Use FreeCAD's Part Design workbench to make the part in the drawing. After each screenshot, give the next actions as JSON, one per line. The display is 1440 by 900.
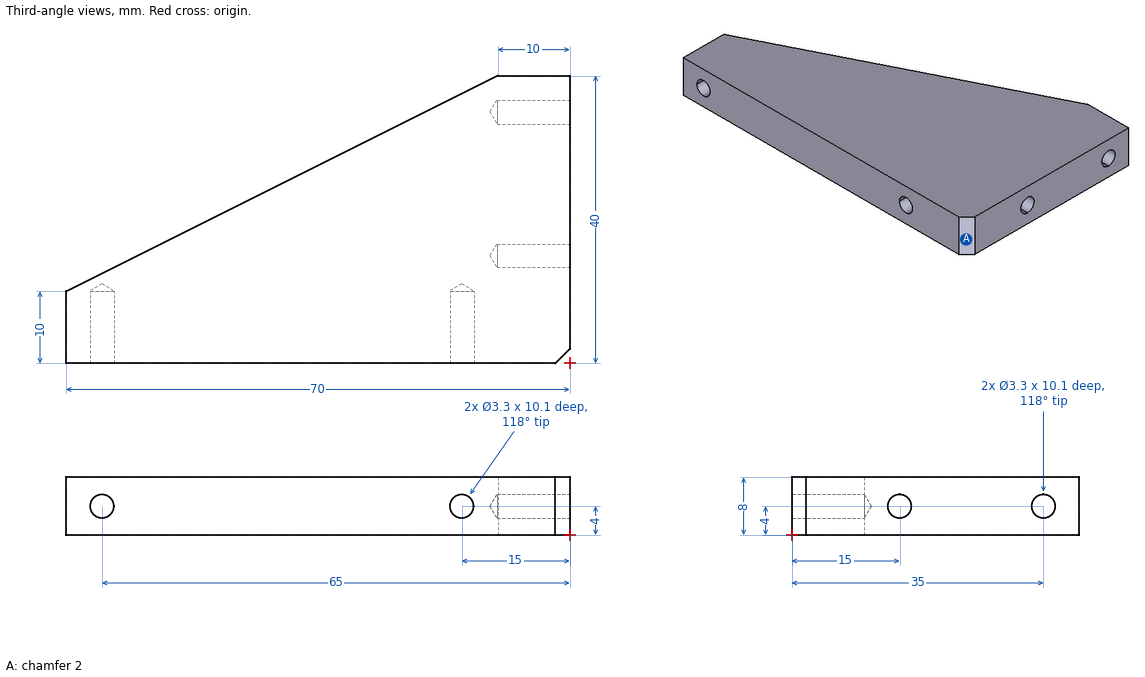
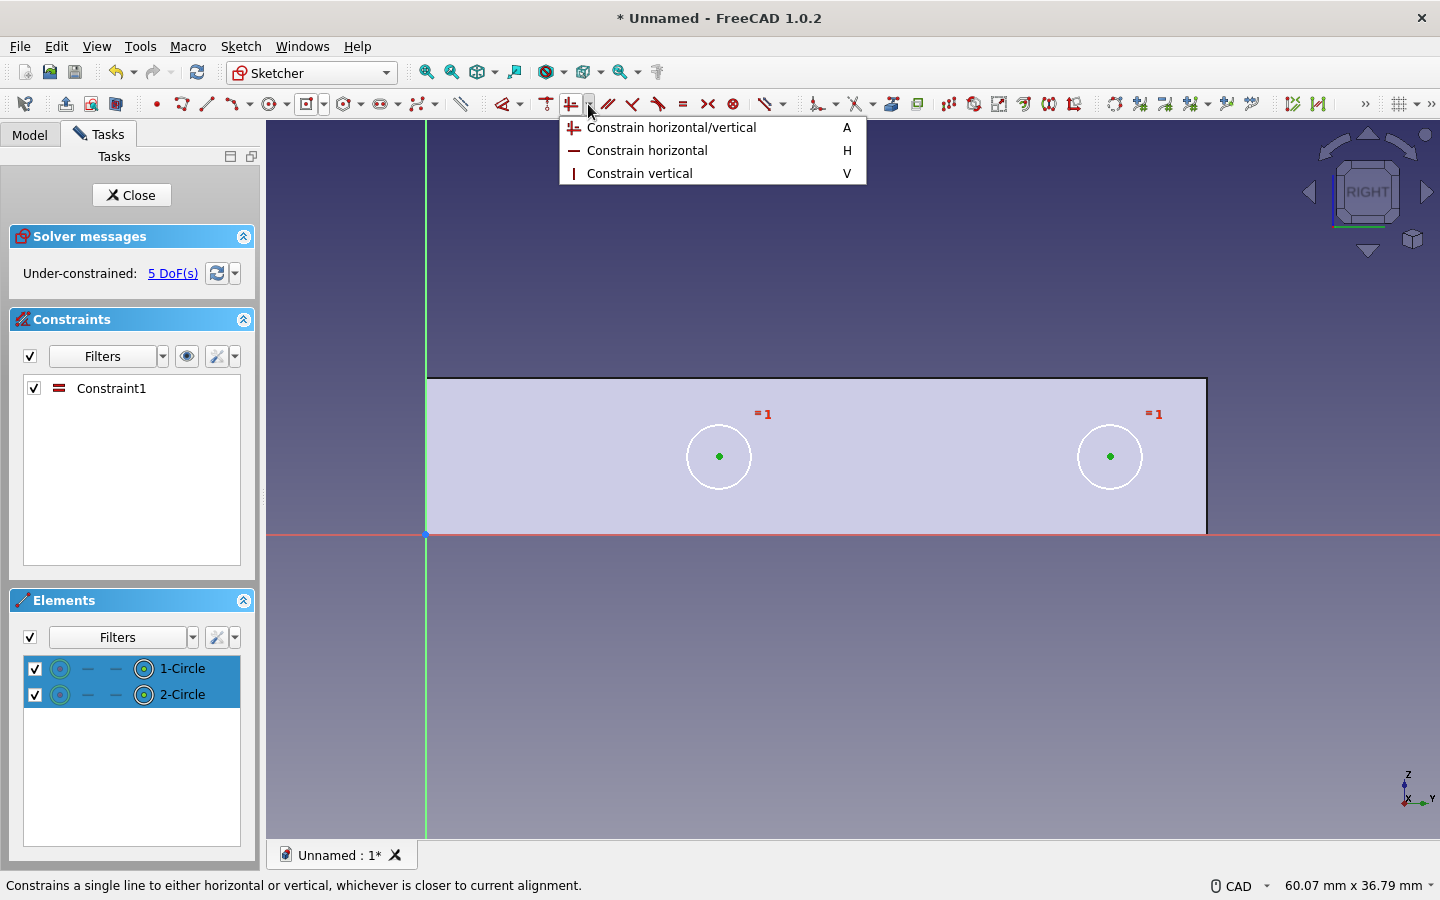
{"action": "left_click", "coordinate": [713, 150]}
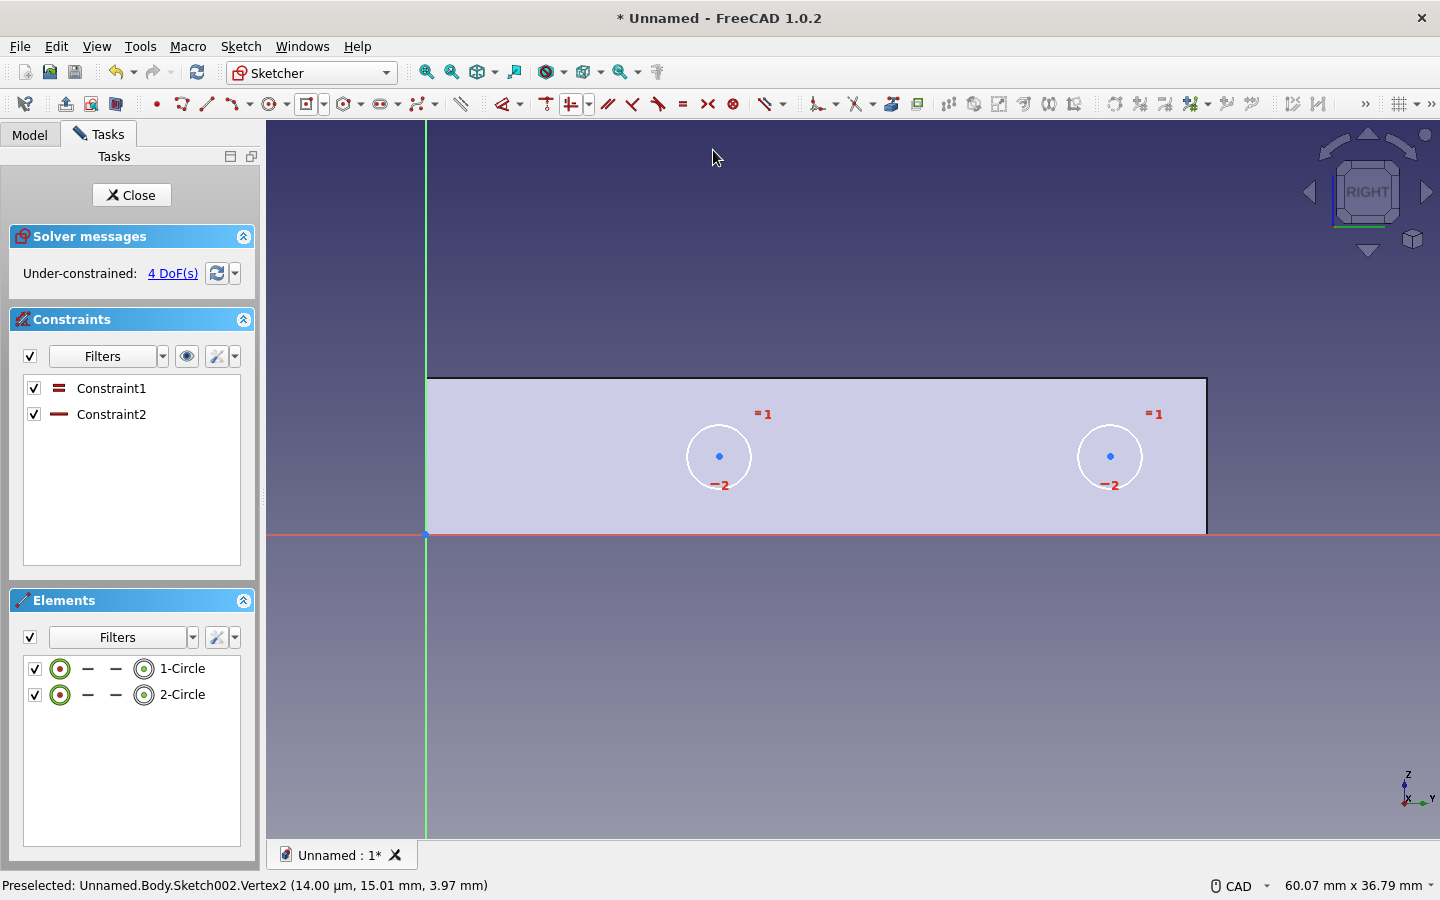
{"action": "left_click", "coordinate": [502, 104]}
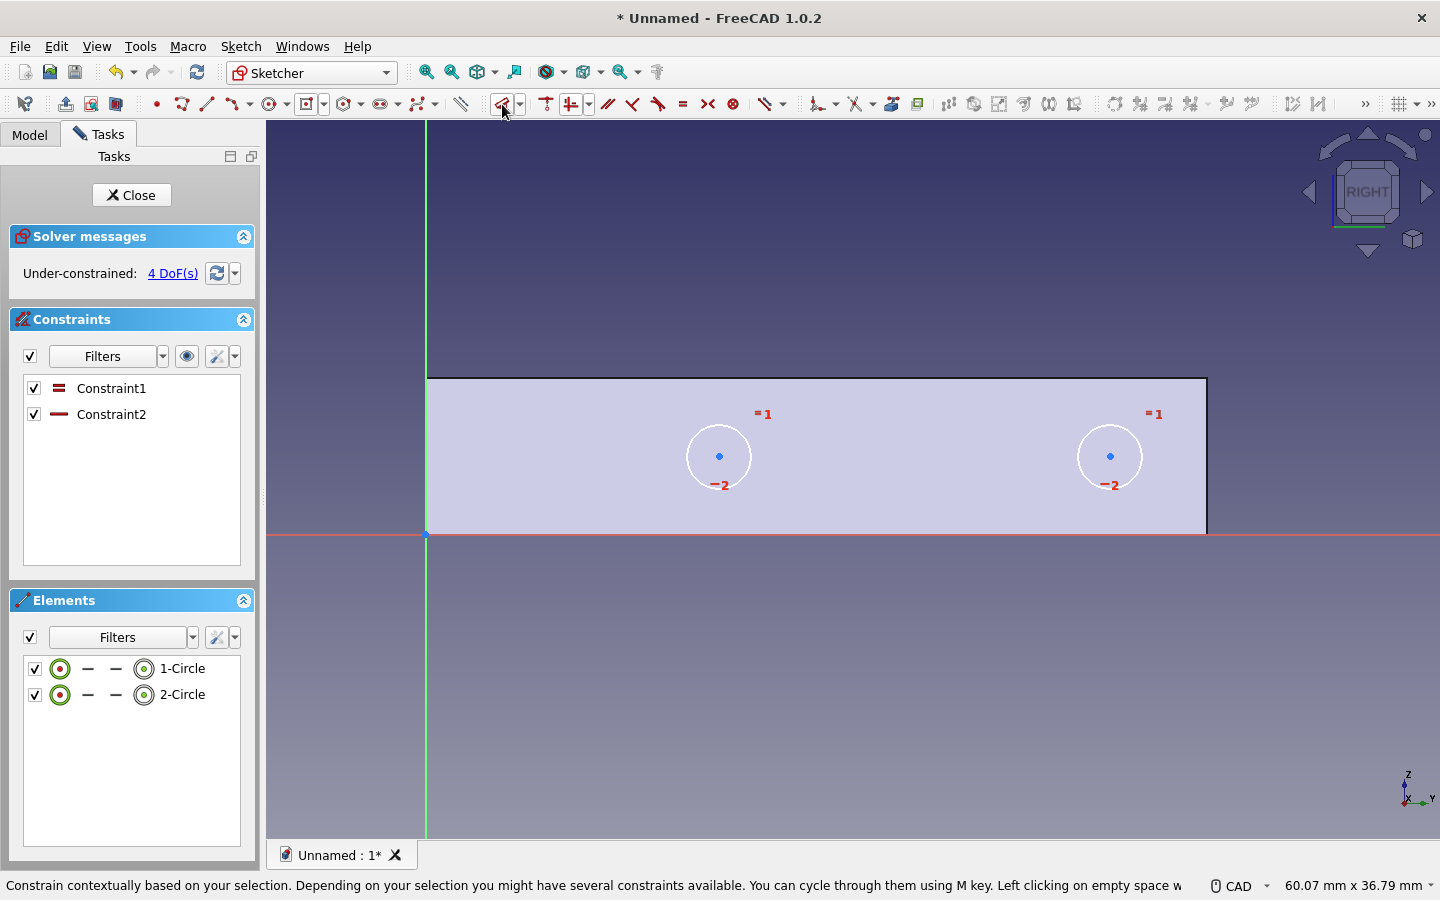
{"action": "left_click", "coordinate": [1132, 434]}
{"action": "left_click", "coordinate": [1154, 411]}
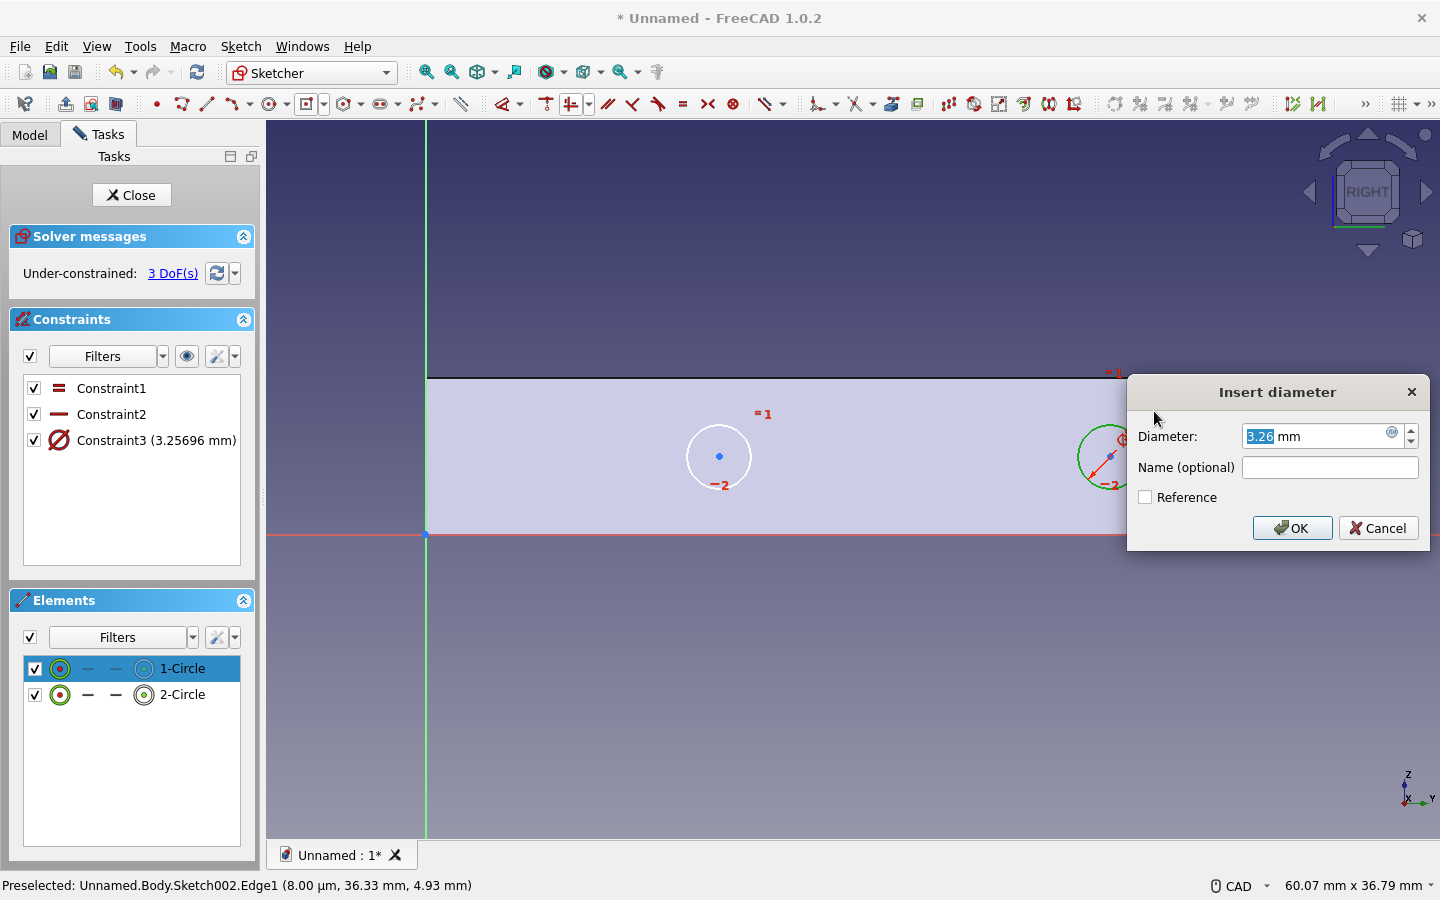
{"action": "type", "text": "3.3"}
{"action": "key", "text": "Return"}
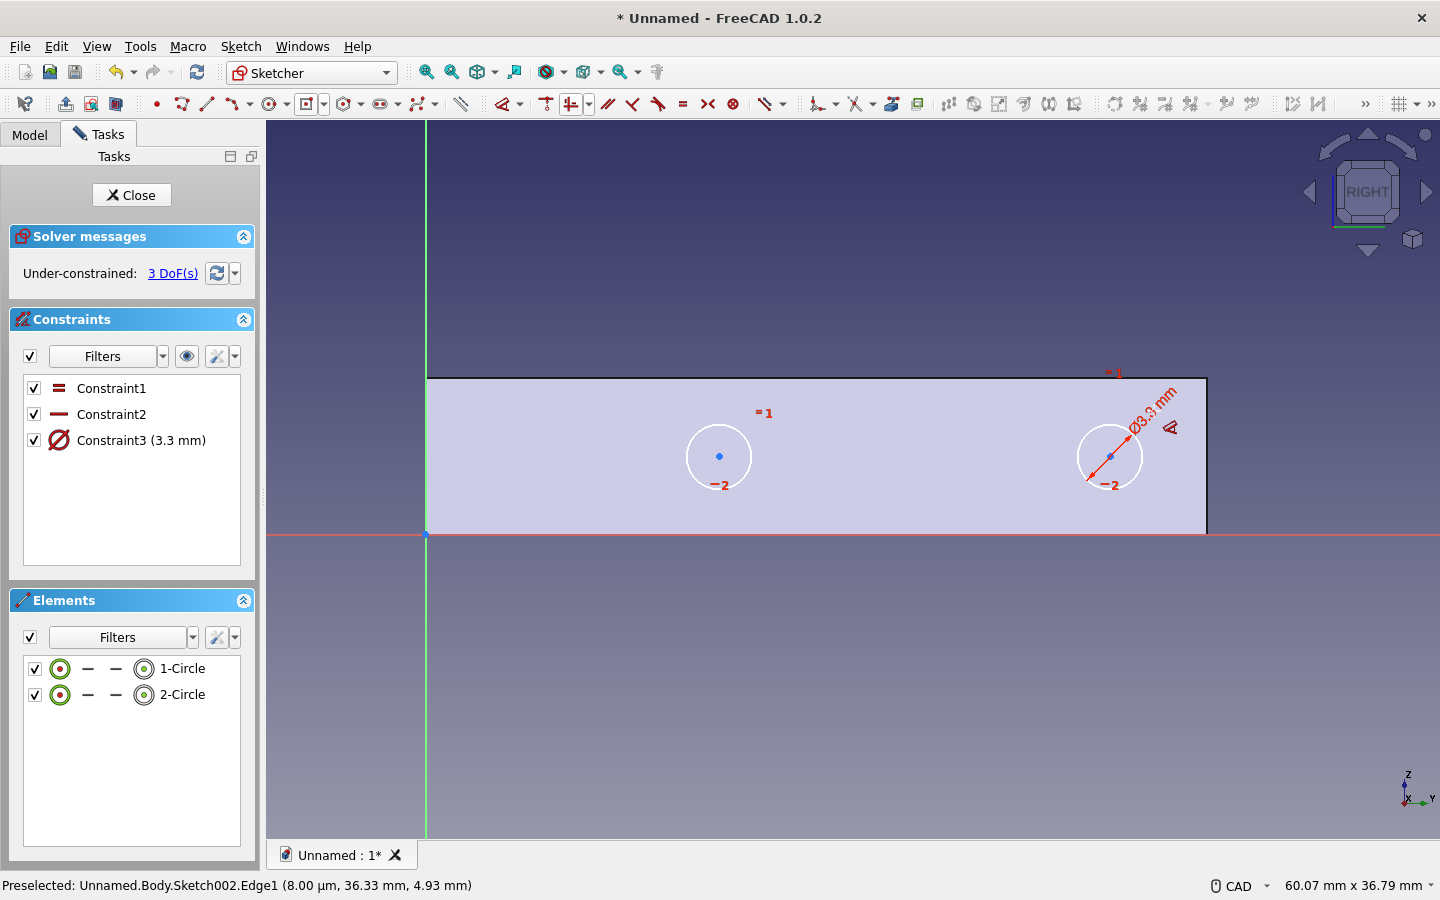
{"action": "left_click", "coordinate": [1110, 457]}
{"action": "left_click", "coordinate": [392, 496]}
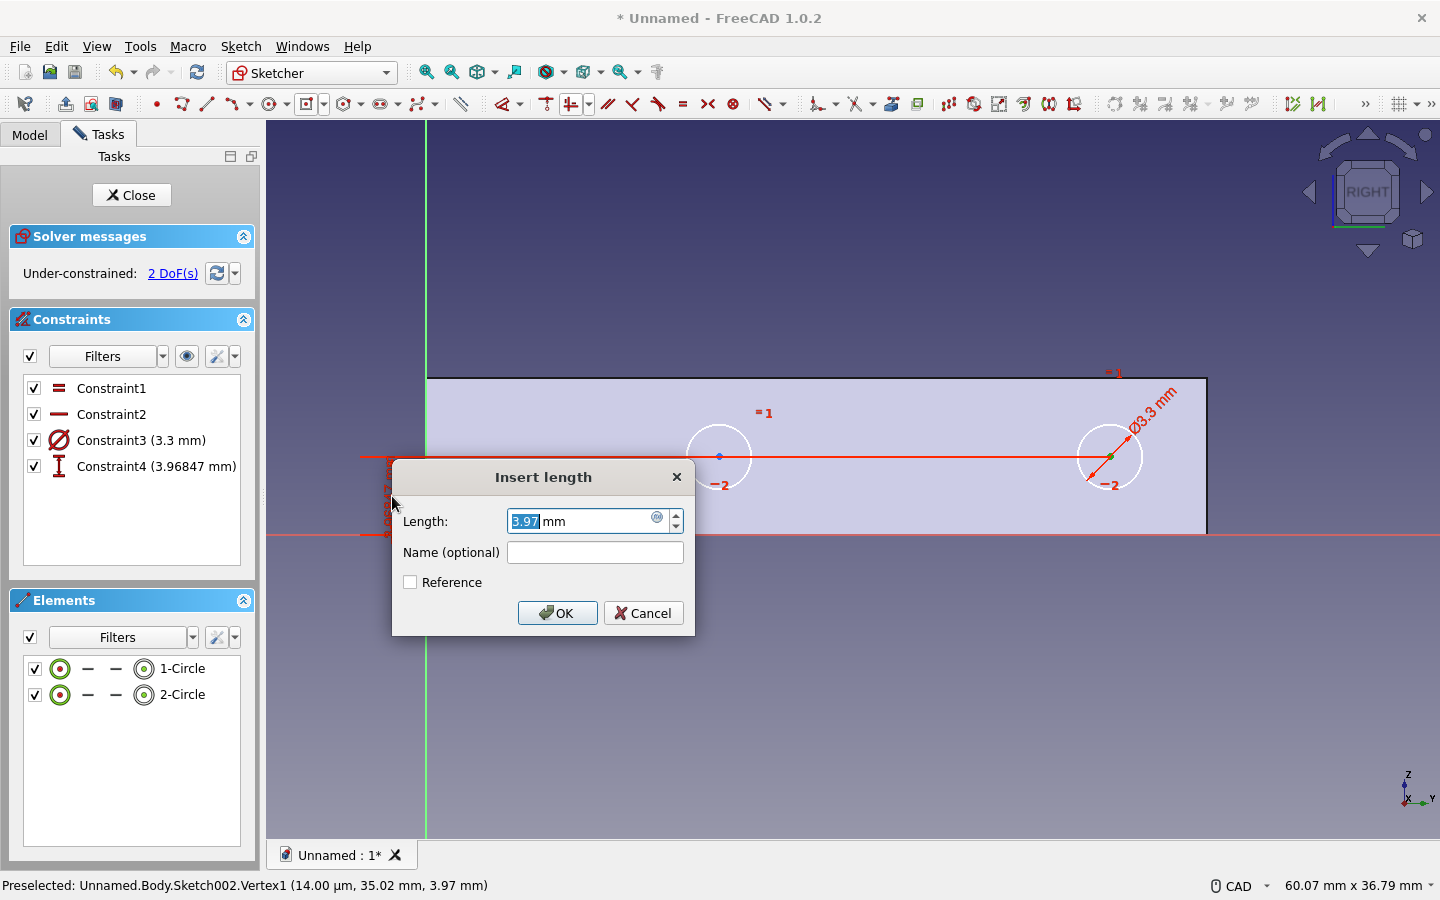
{"action": "type", "text": "4"}
{"action": "key", "text": "Return"}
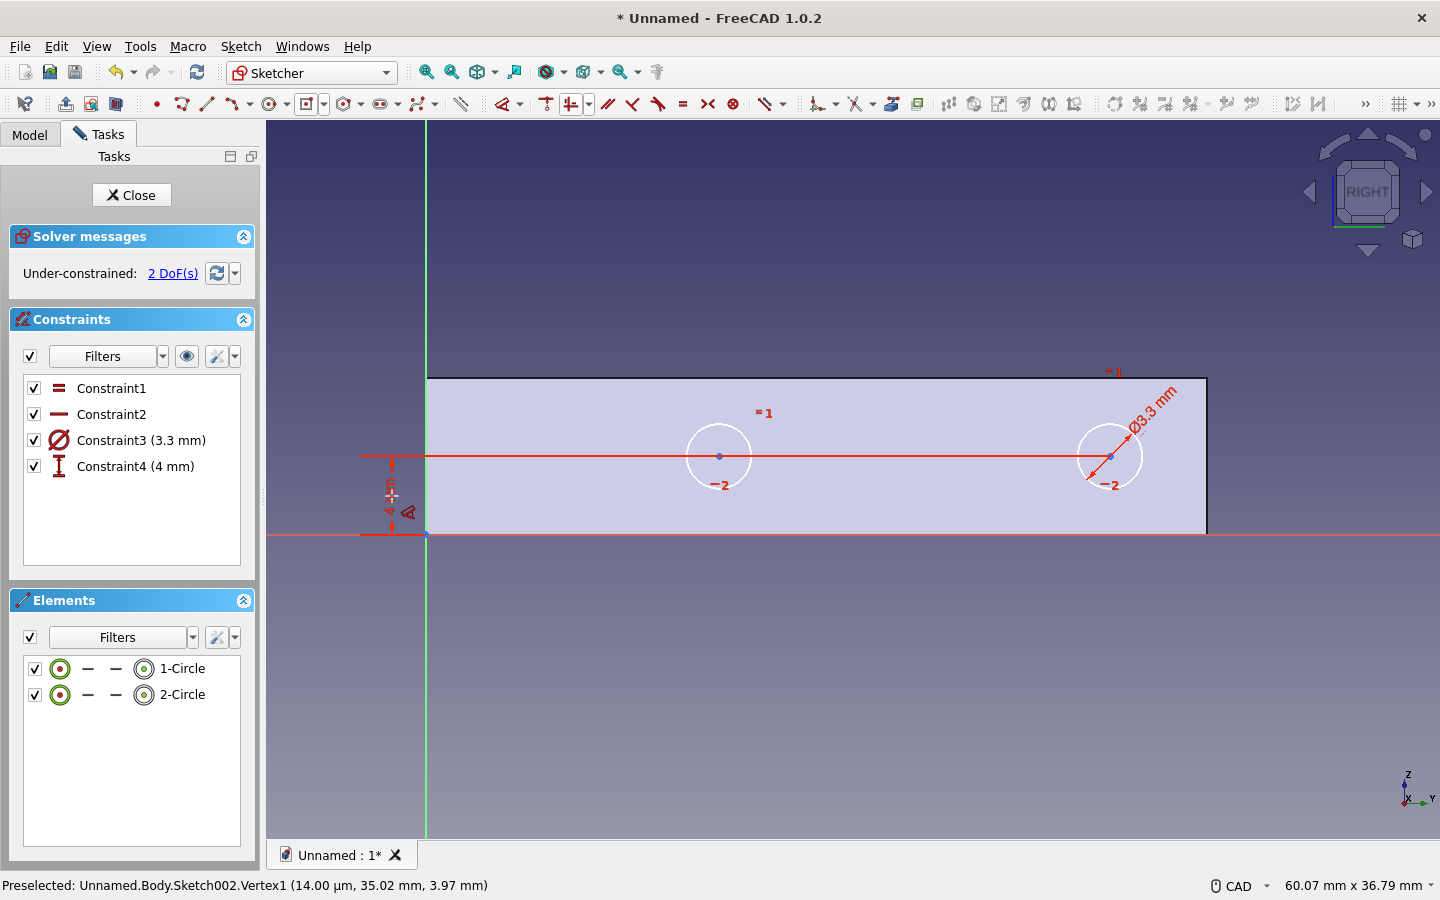
{"action": "left_click", "coordinate": [1110, 456]}
{"action": "left_click", "coordinate": [768, 569]}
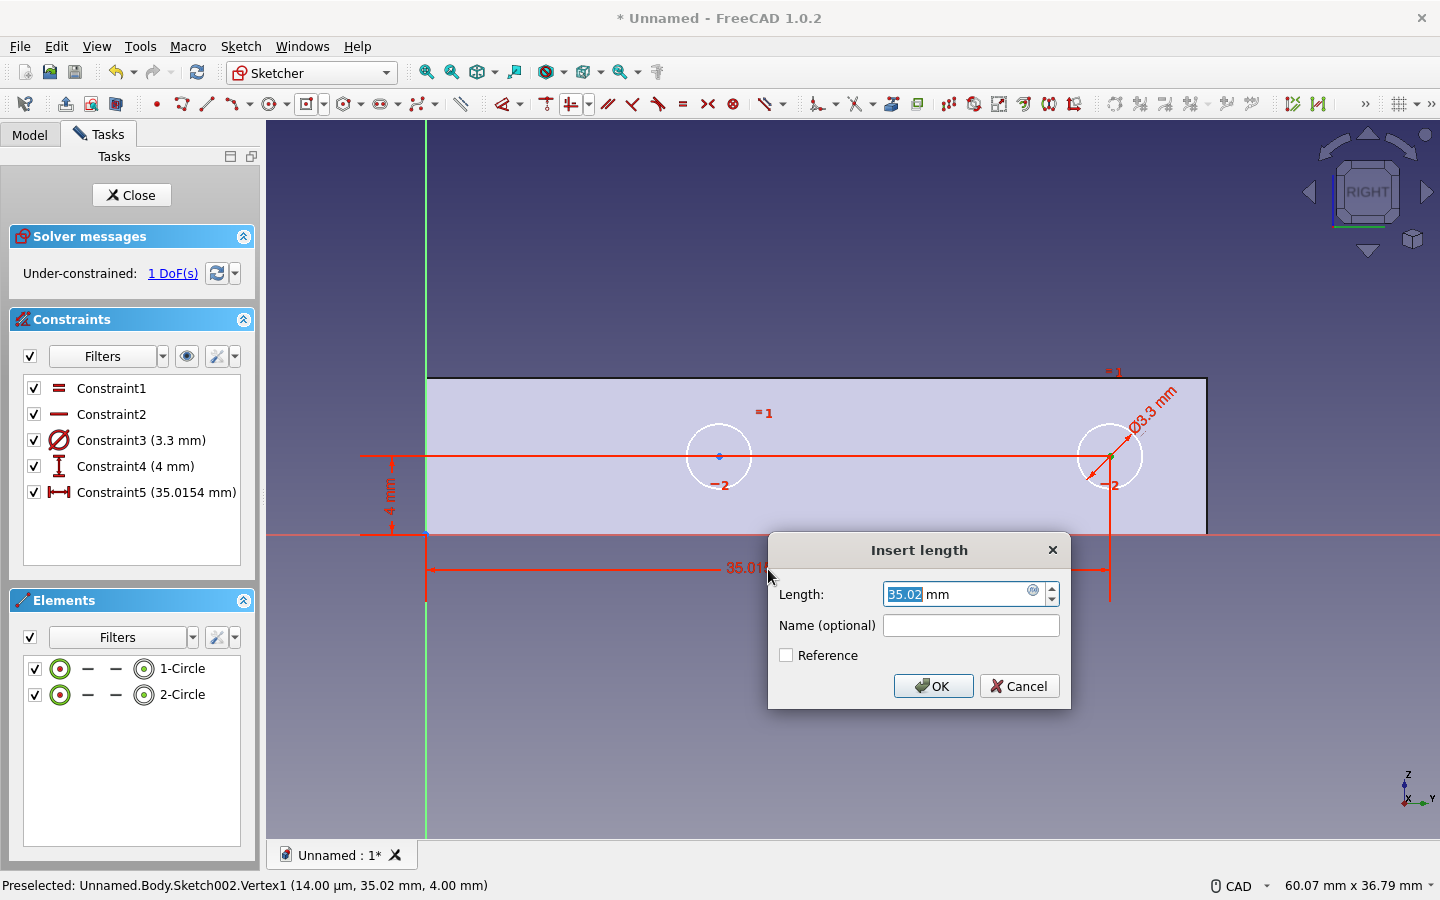
{"action": "type", "text": "35"}
{"action": "key", "text": "Return"}